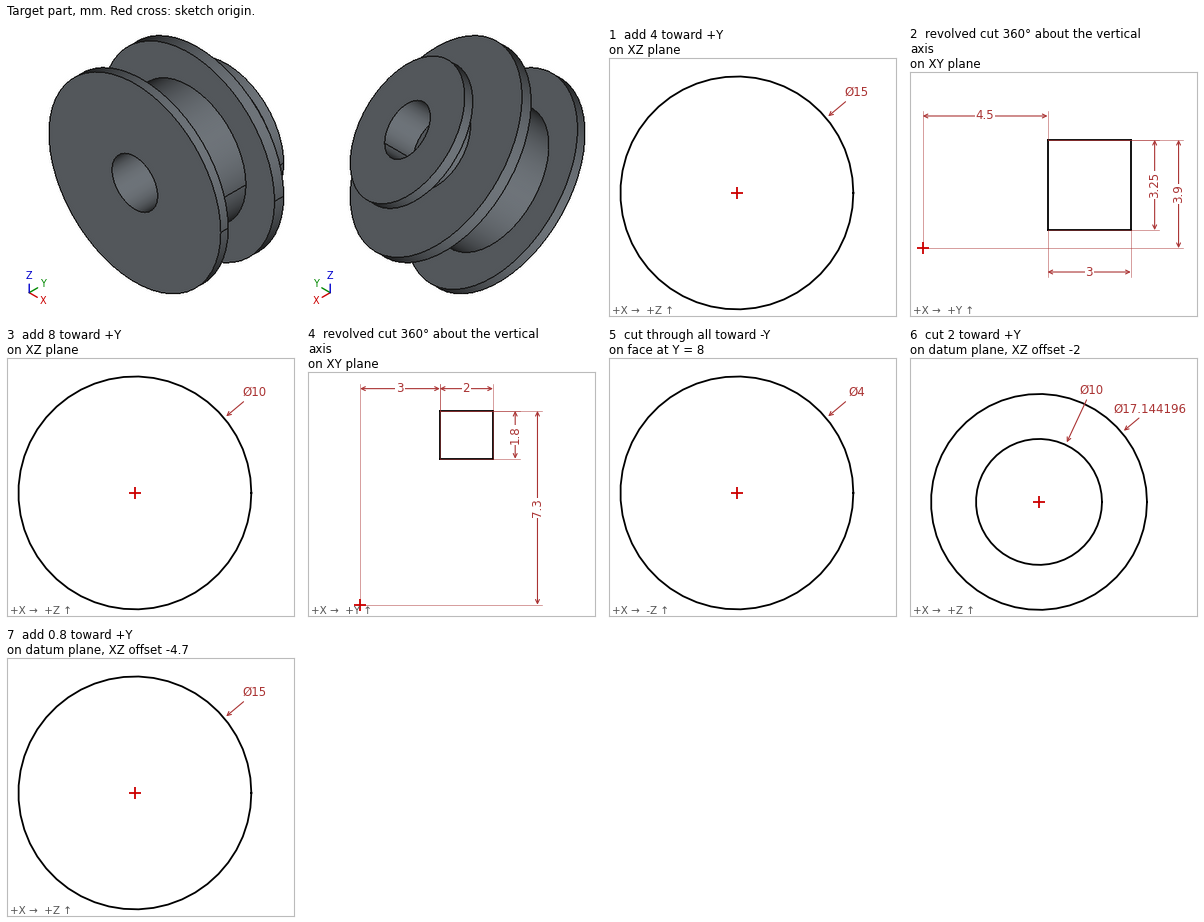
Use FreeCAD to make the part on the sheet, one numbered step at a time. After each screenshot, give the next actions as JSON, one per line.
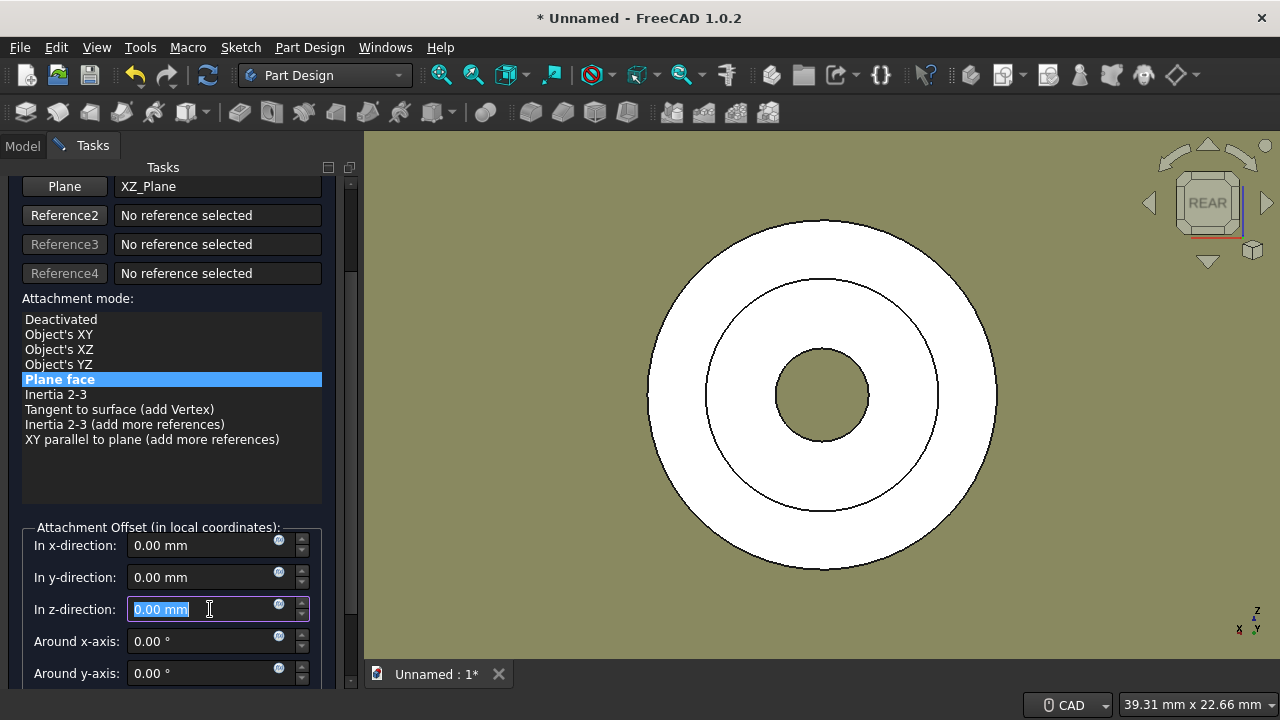
{"action": "type", "text": "-2"}
{"action": "key", "text": "Tab"}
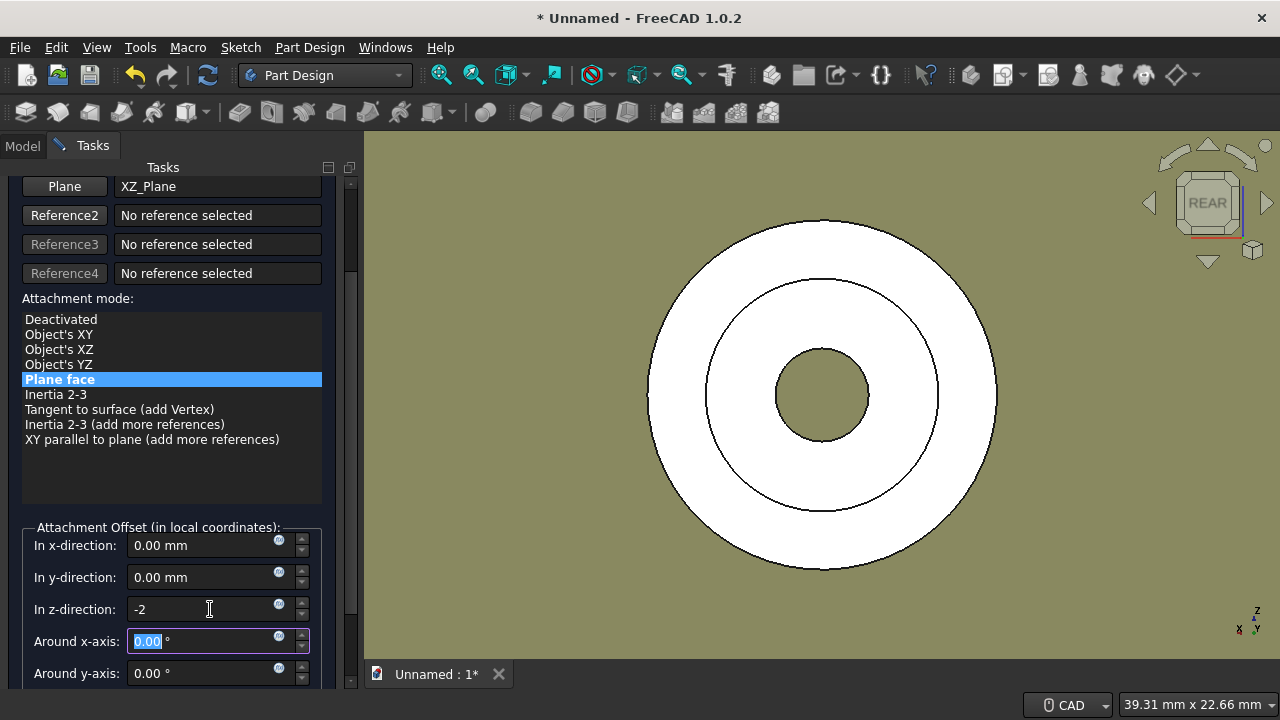
{"action": "scroll", "coordinate": [351, 432], "scroll_direction": "up", "scroll_amount": 3}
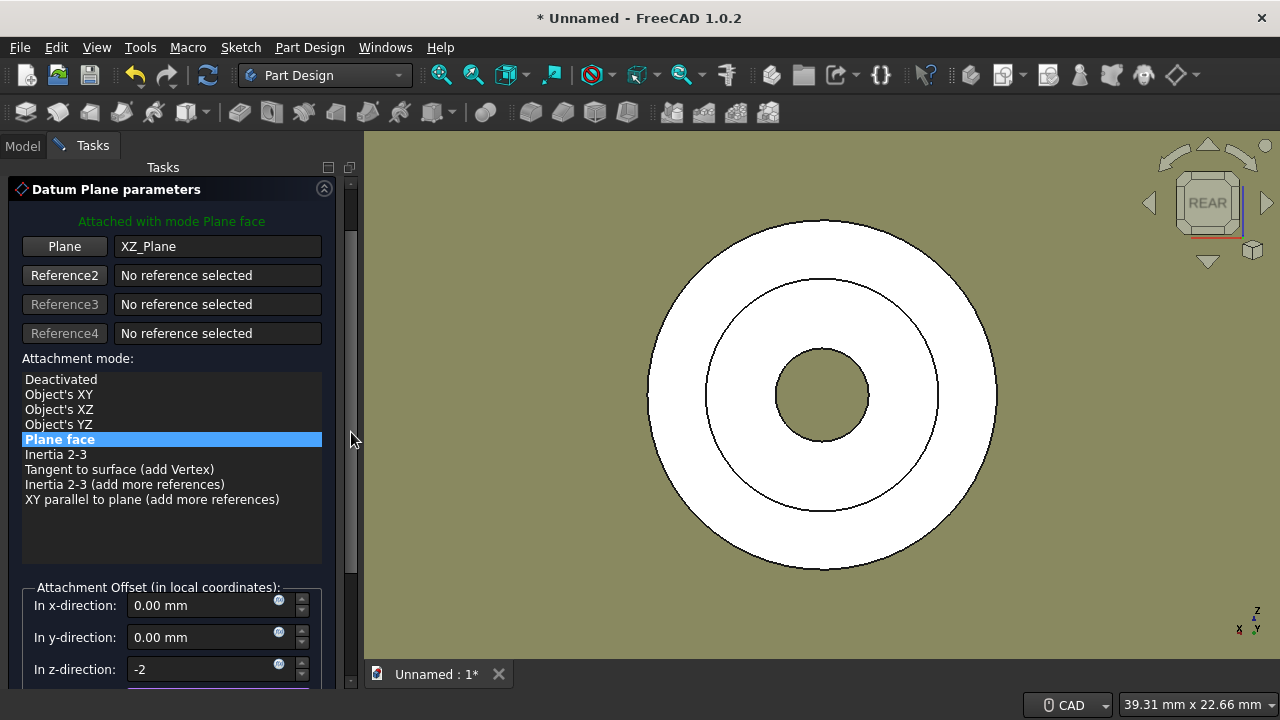
{"action": "left_click", "coordinate": [124, 206]}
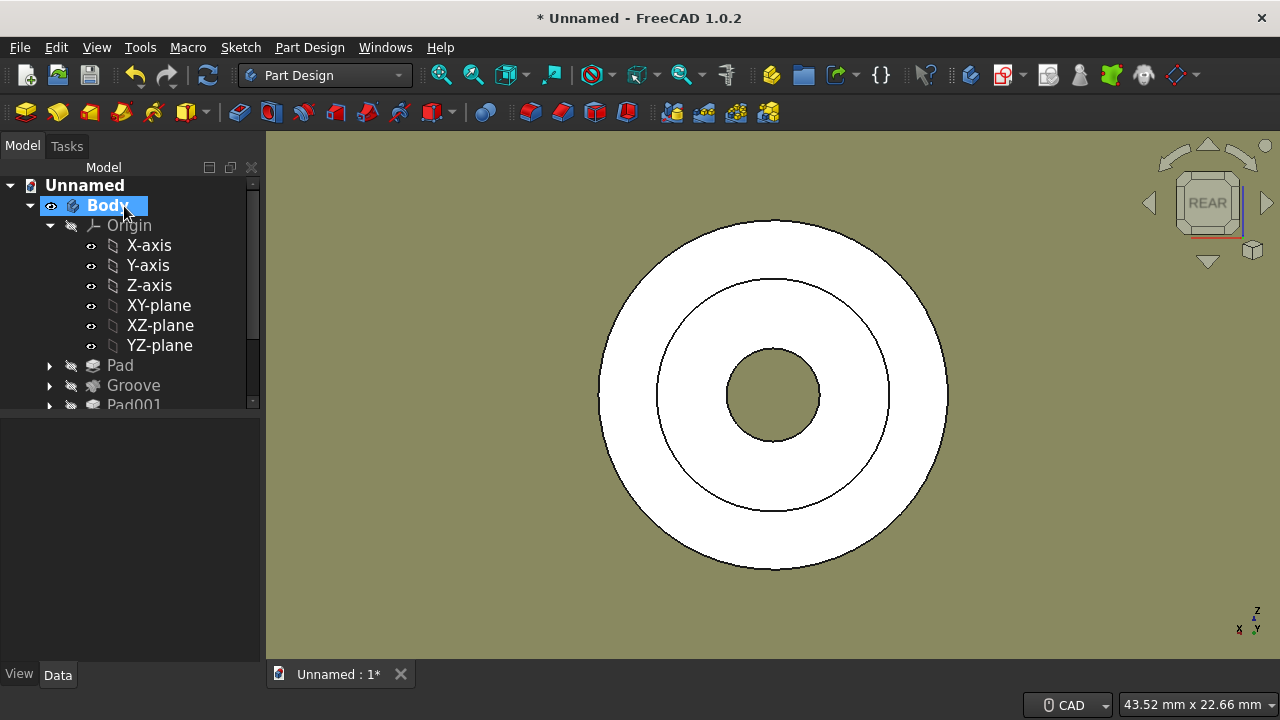
{"action": "scroll", "coordinate": [100, 301], "scroll_direction": "down", "scroll_amount": 3}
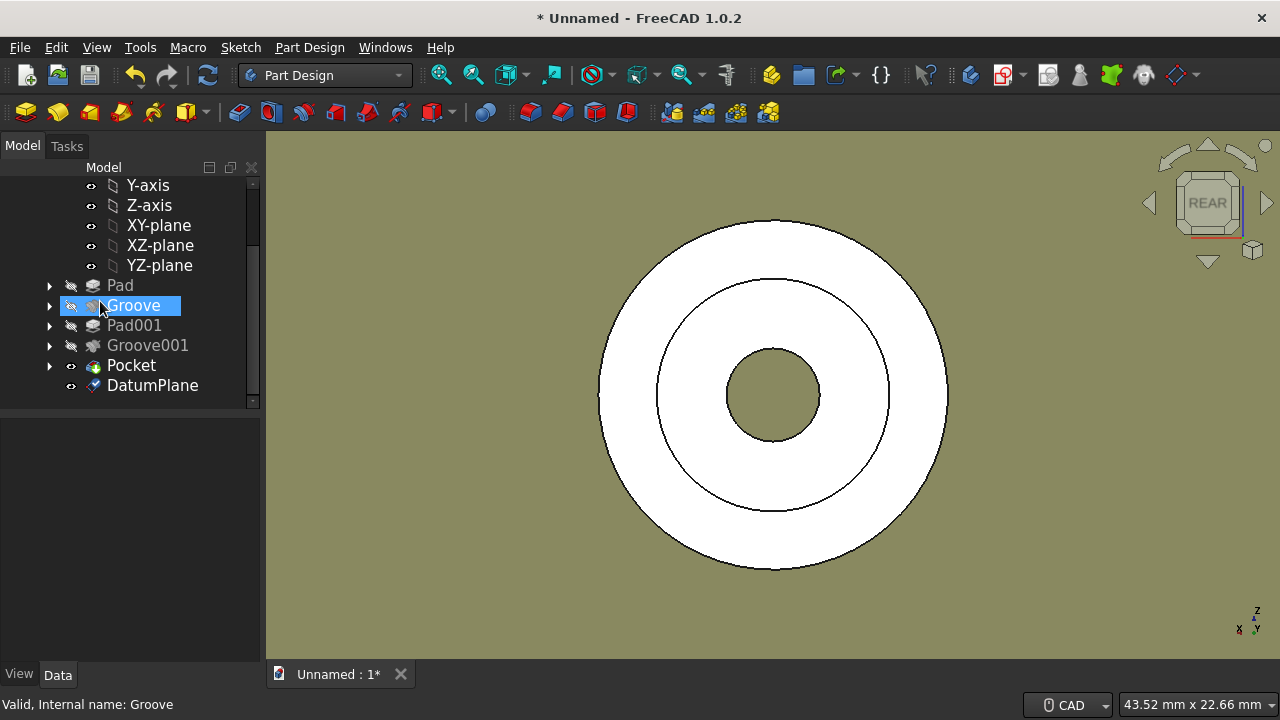
{"action": "left_click", "coordinate": [116, 386]}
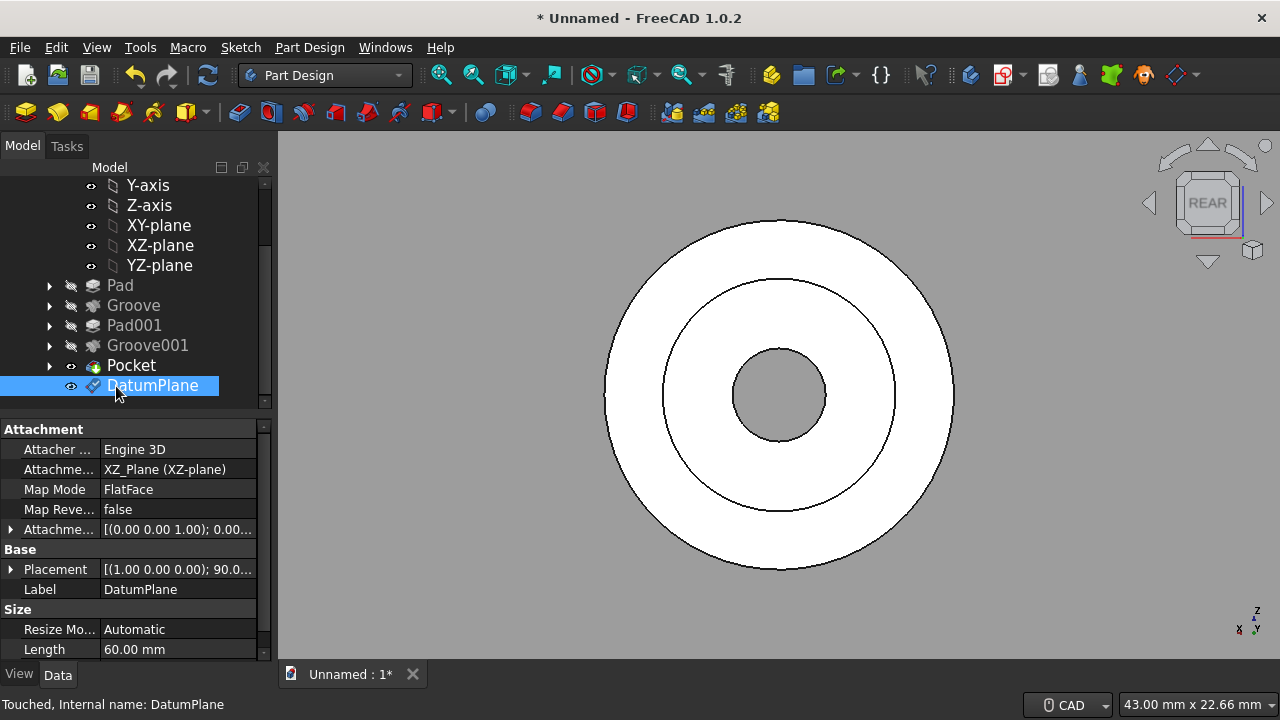
{"action": "left_click", "coordinate": [1004, 76]}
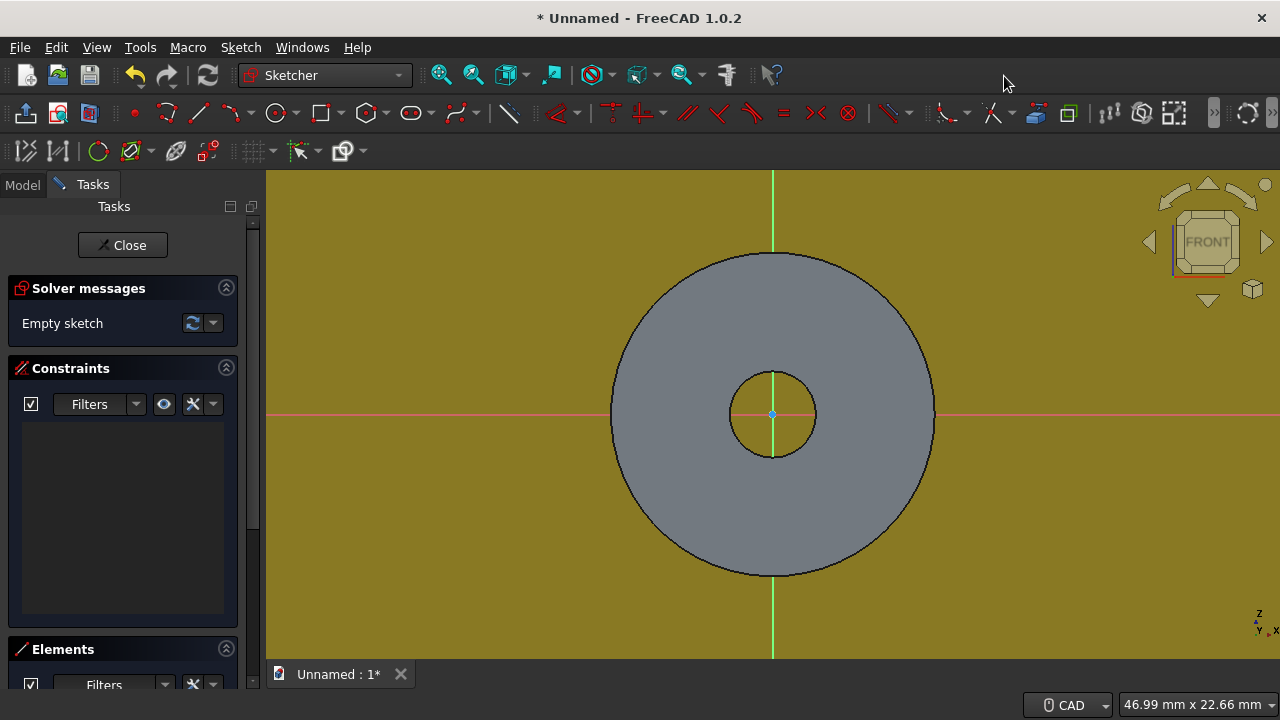
{"action": "left_click", "coordinate": [90, 114]}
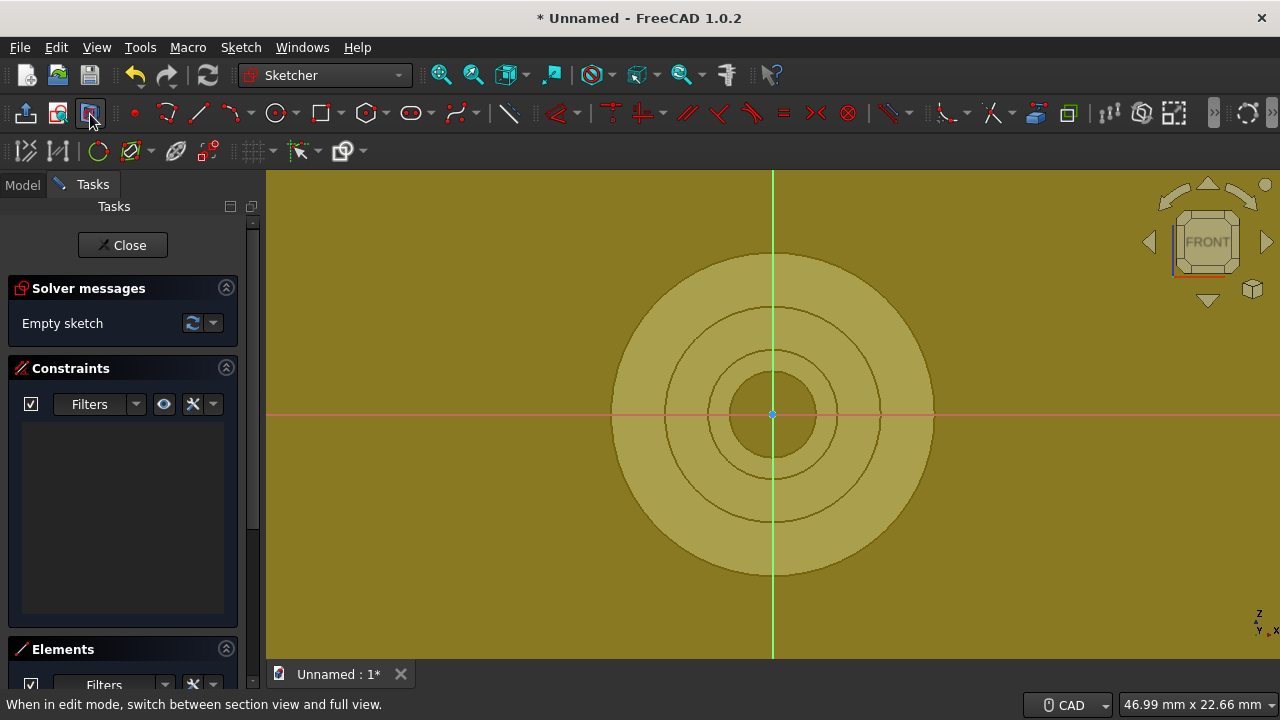
{"action": "key", "text": "g c"}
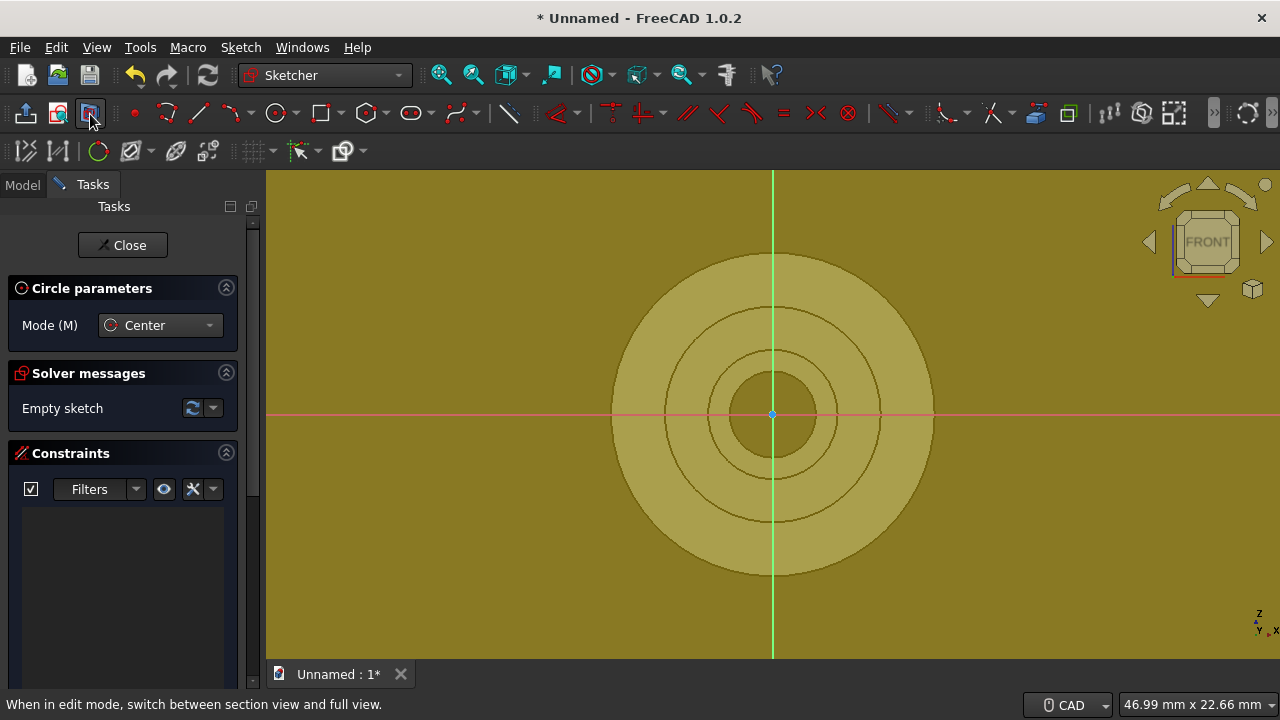
{"action": "left_click", "coordinate": [773, 415]}
{"action": "left_click", "coordinate": [904, 284]}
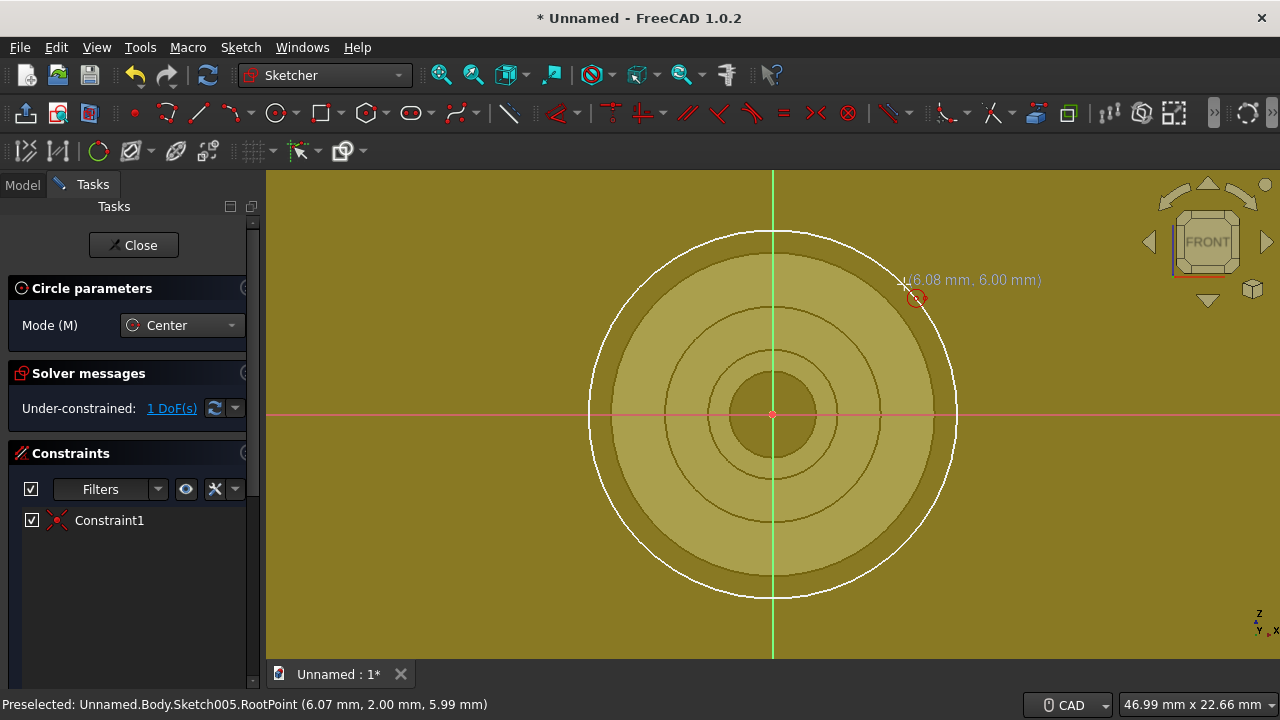
{"action": "left_click", "coordinate": [773, 415]}
{"action": "left_click", "coordinate": [849, 338]}
{"action": "key", "text": "Escape"}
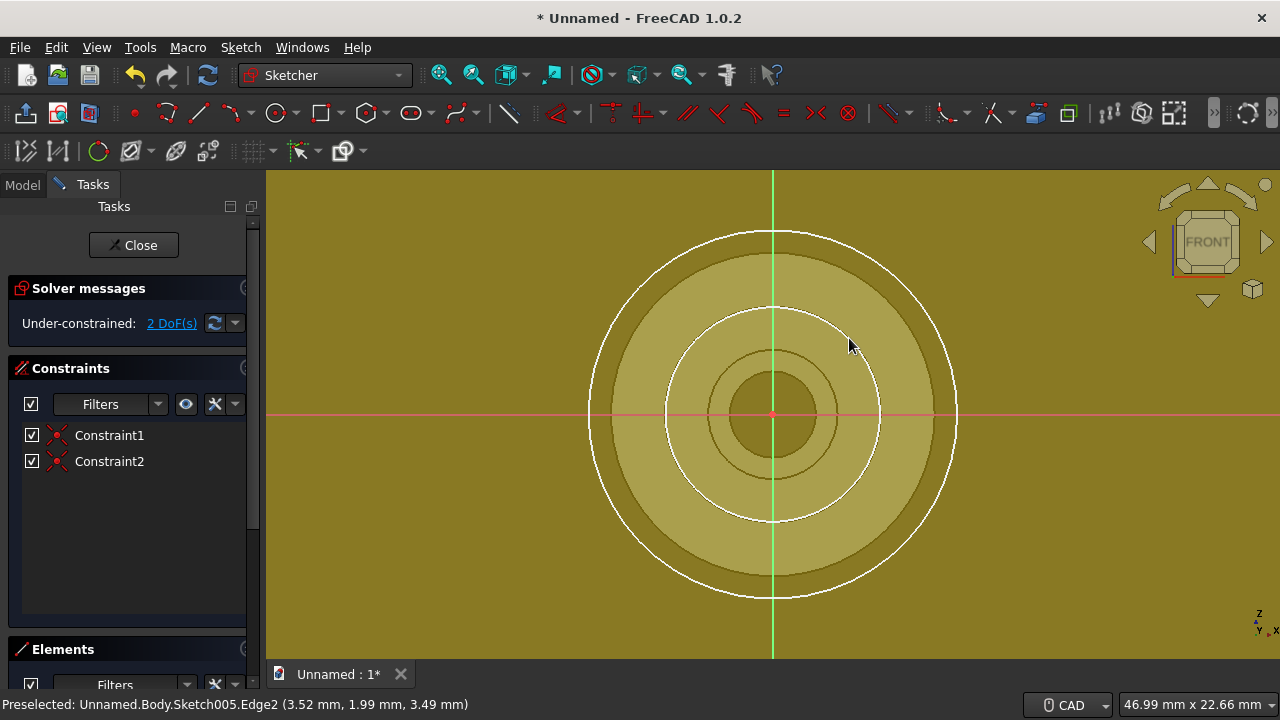
{"action": "left_click", "coordinate": [556, 114]}